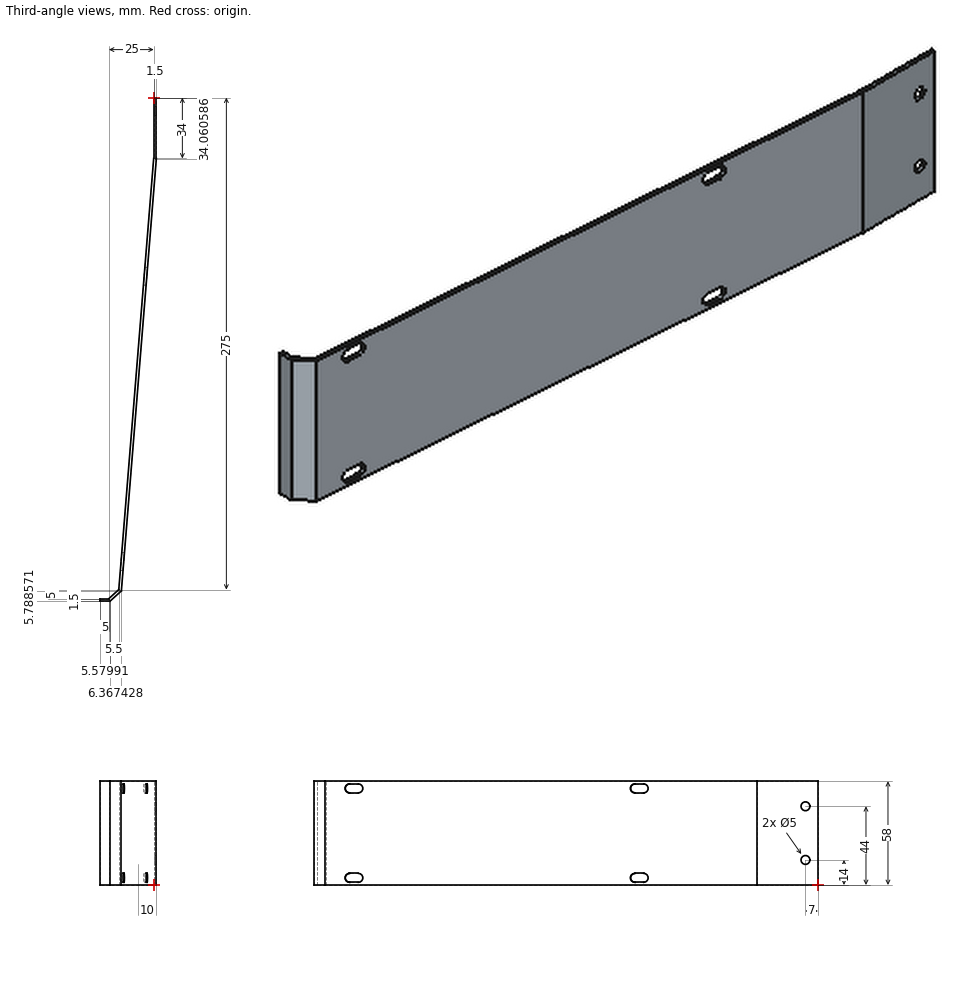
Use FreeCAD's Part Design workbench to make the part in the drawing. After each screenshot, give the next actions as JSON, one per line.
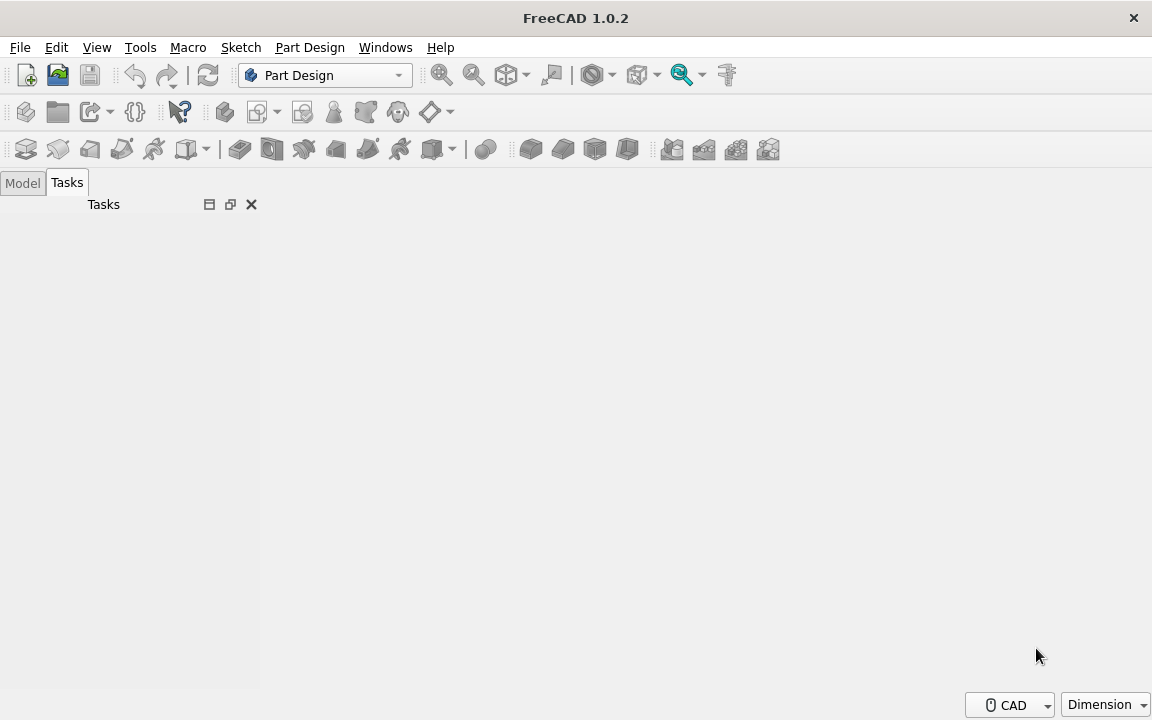
{"action": "left_click", "coordinate": [26, 76]}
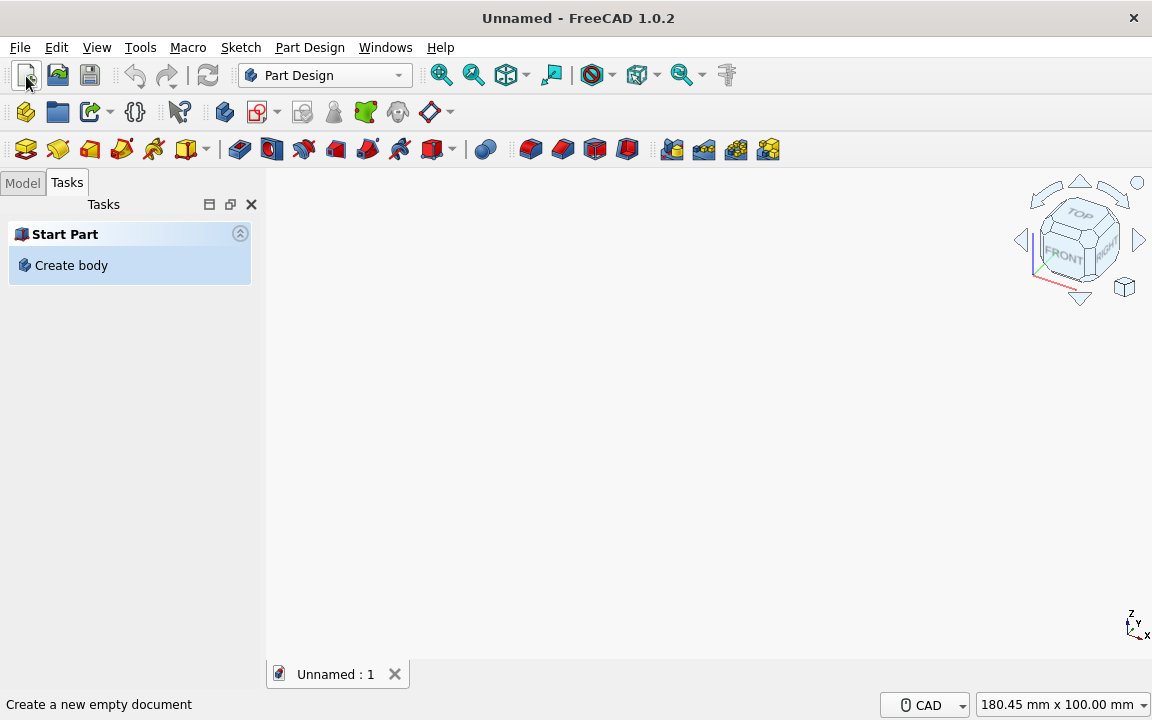
{"action": "left_click", "coordinate": [258, 112]}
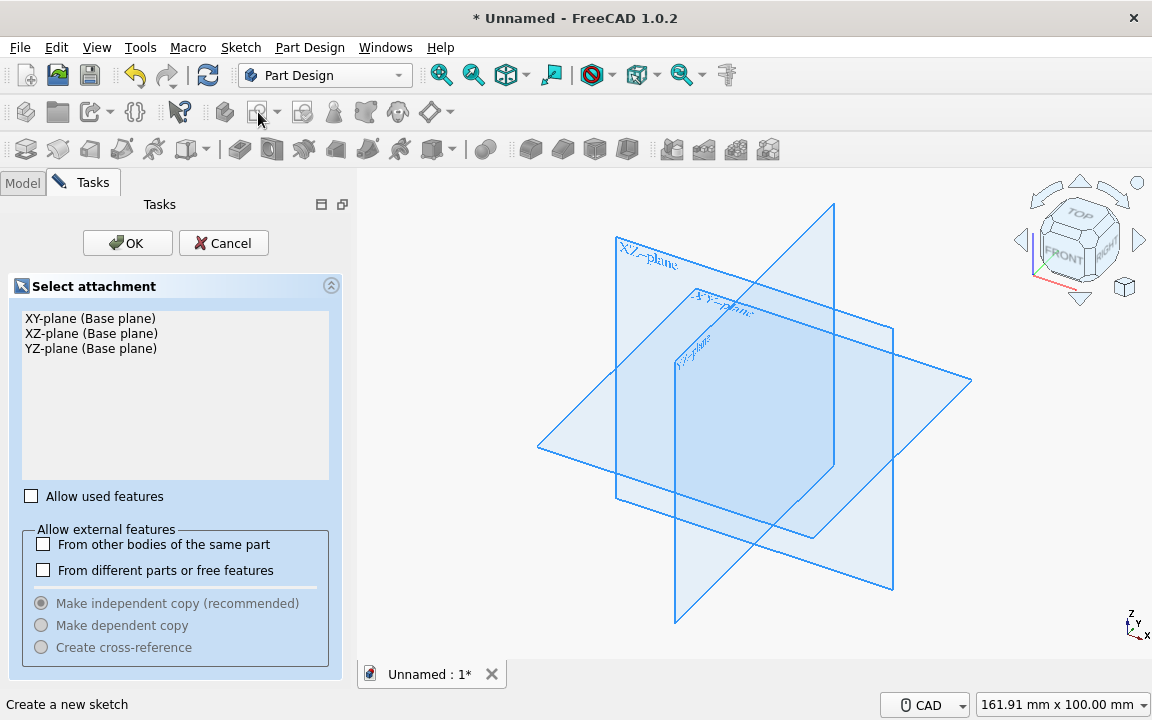
{"action": "left_click", "coordinate": [82, 318]}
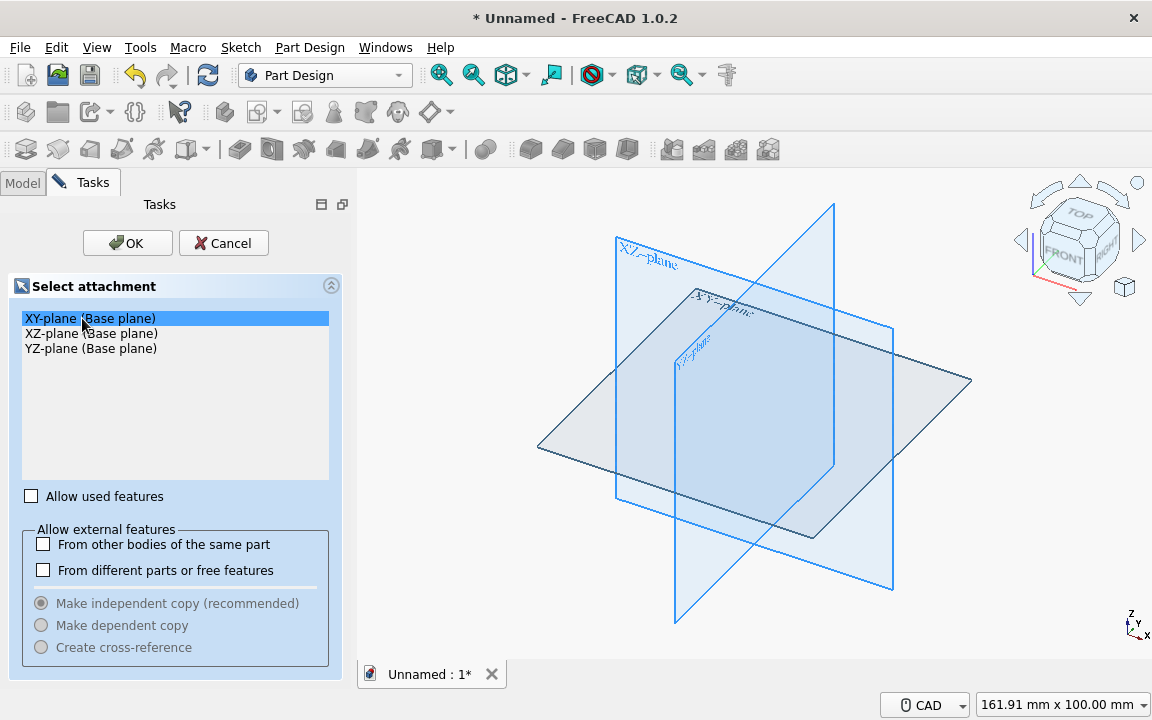
{"action": "left_click", "coordinate": [128, 243]}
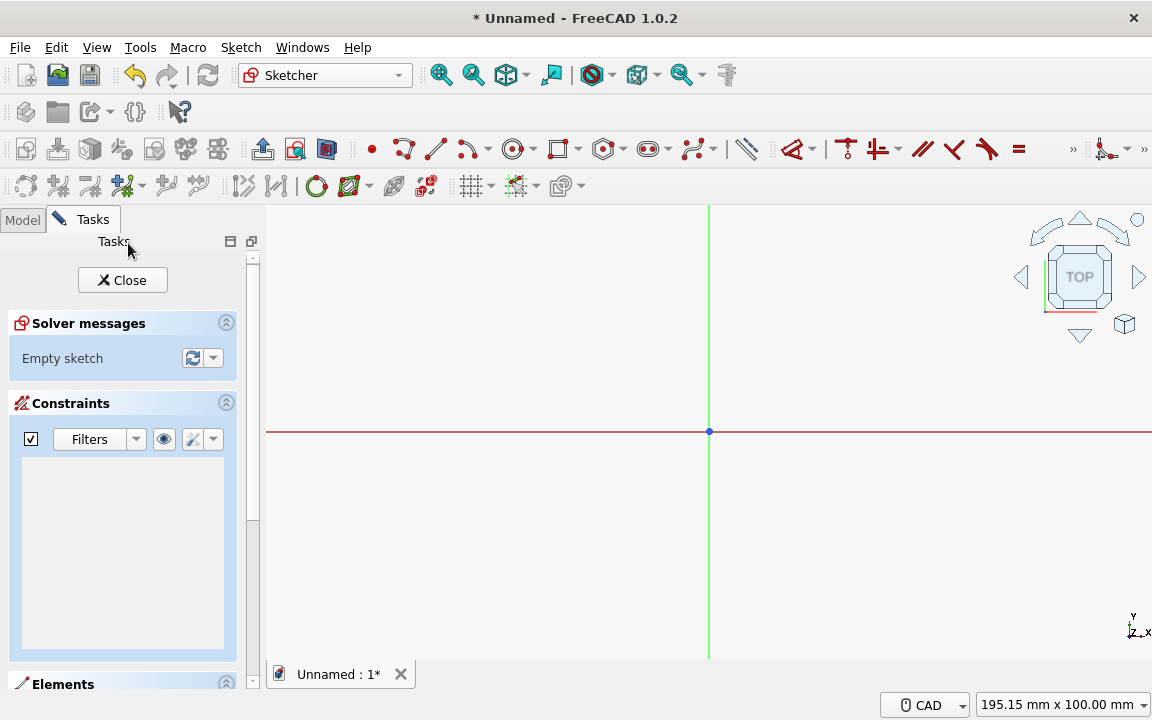
{"action": "scroll", "coordinate": [640, 270], "scroll_direction": "down", "scroll_amount": 8}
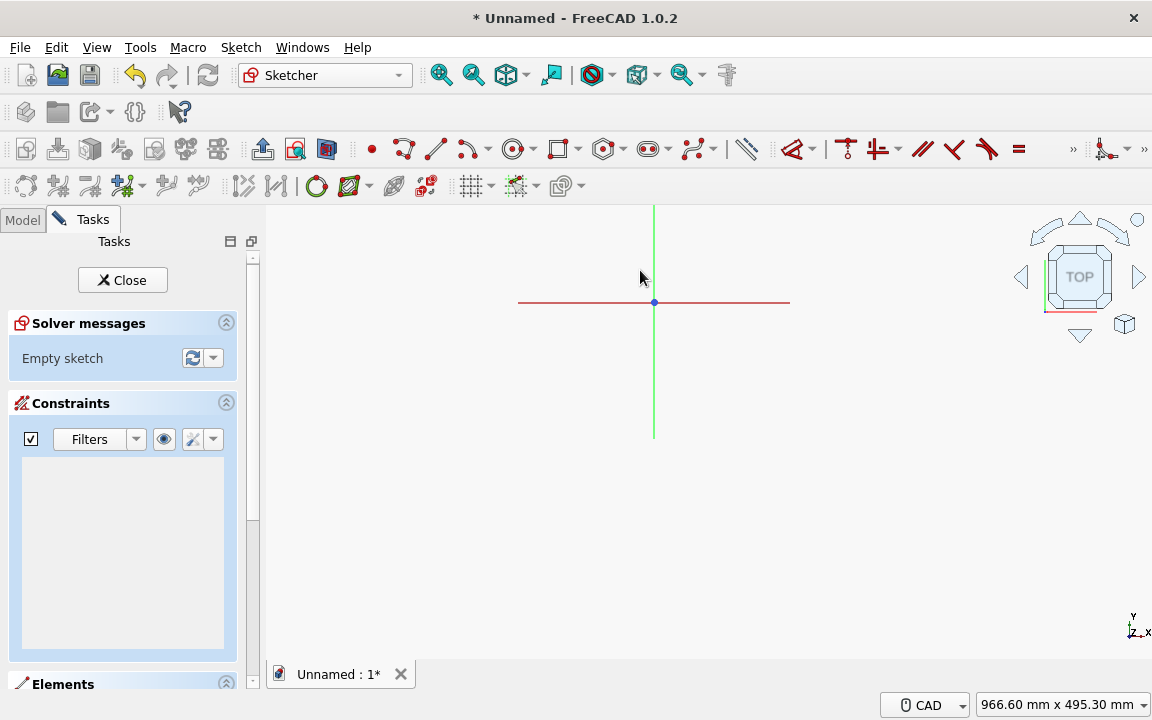
{"action": "left_click", "coordinate": [404, 150]}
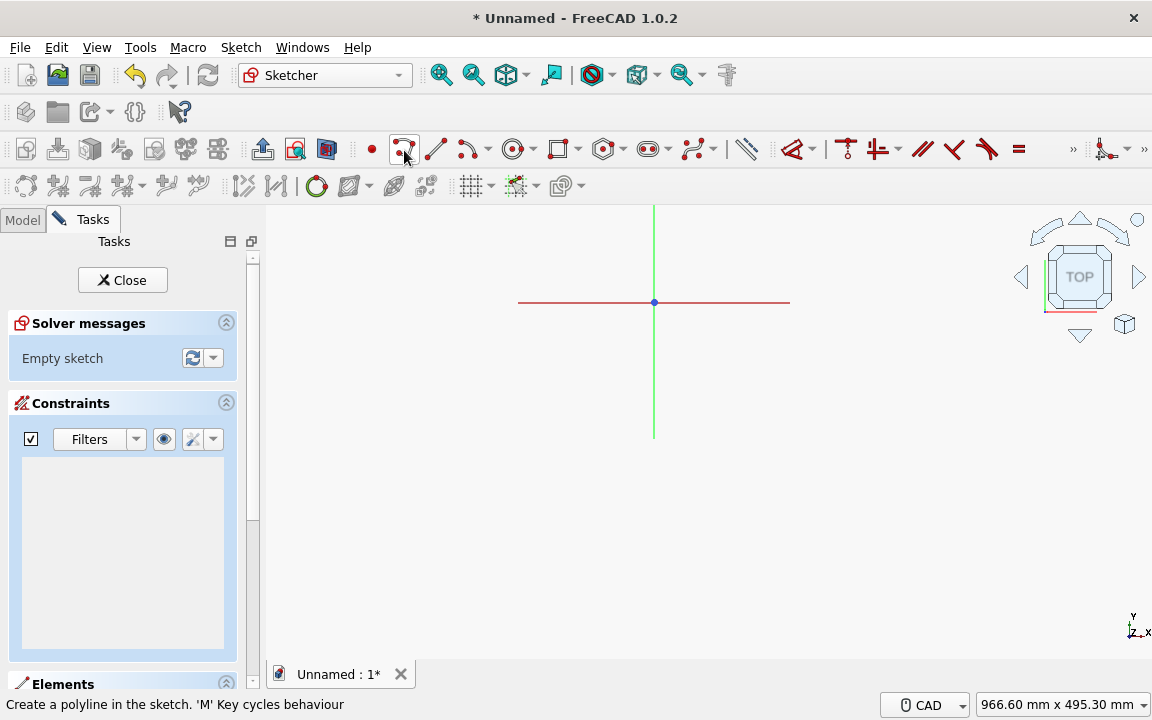
{"action": "left_click", "coordinate": [654, 303]}
{"action": "left_click", "coordinate": [645, 334]}
{"action": "left_click", "coordinate": [636, 555]}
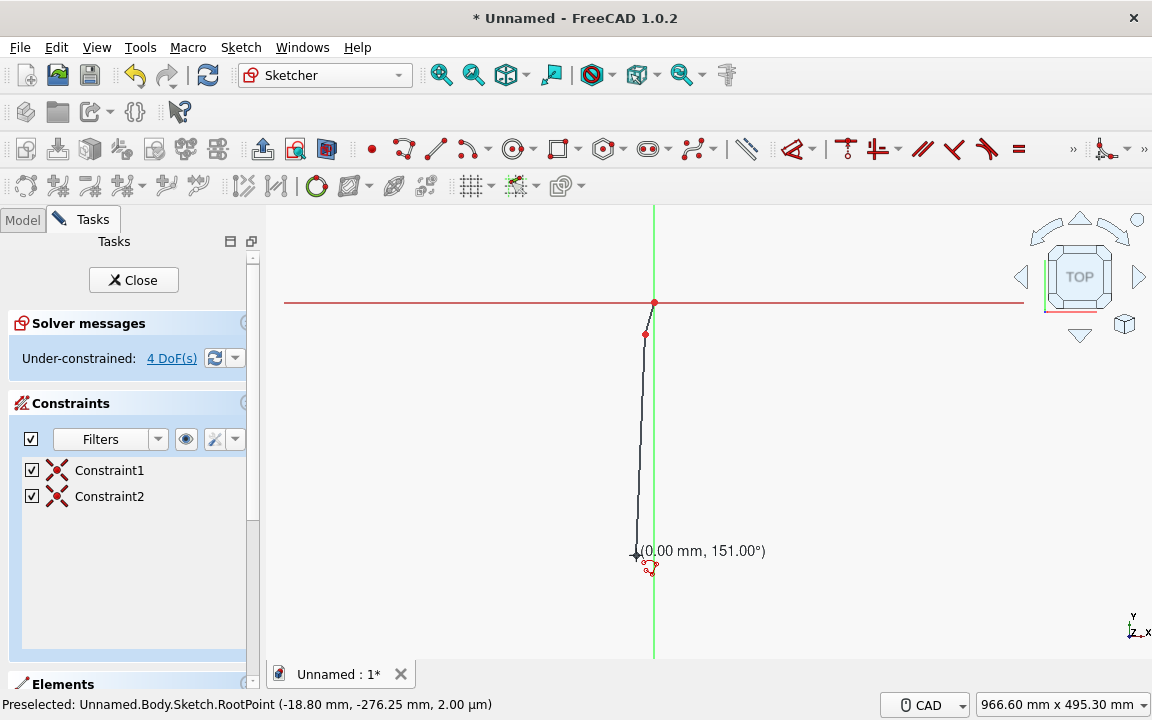
{"action": "scroll", "coordinate": [631, 559], "scroll_direction": "up", "scroll_amount": 5}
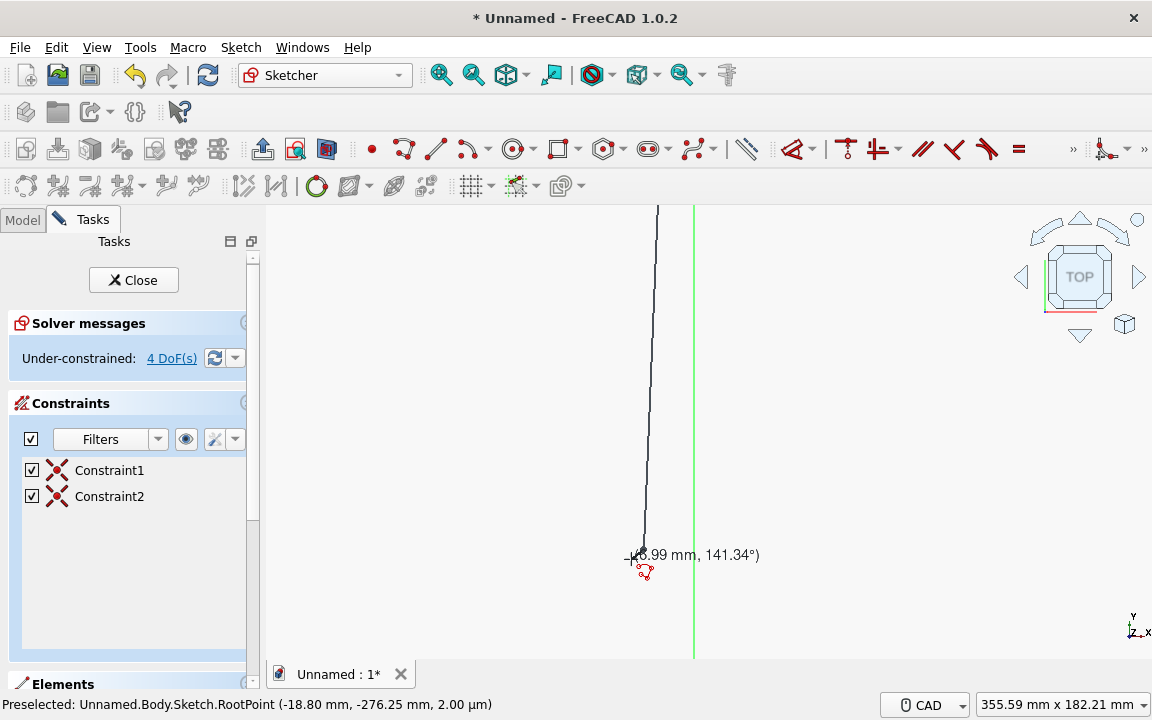
{"action": "left_click", "coordinate": [631, 559]}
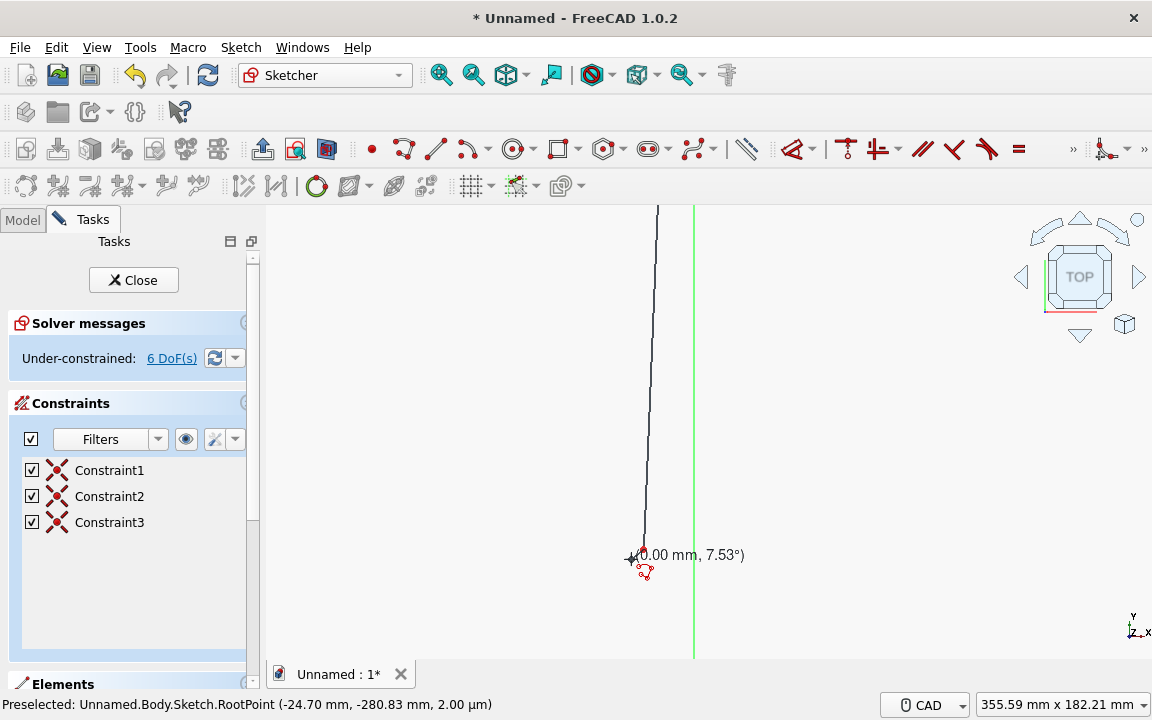
{"action": "scroll", "coordinate": [619, 559], "scroll_direction": "up", "scroll_amount": 2}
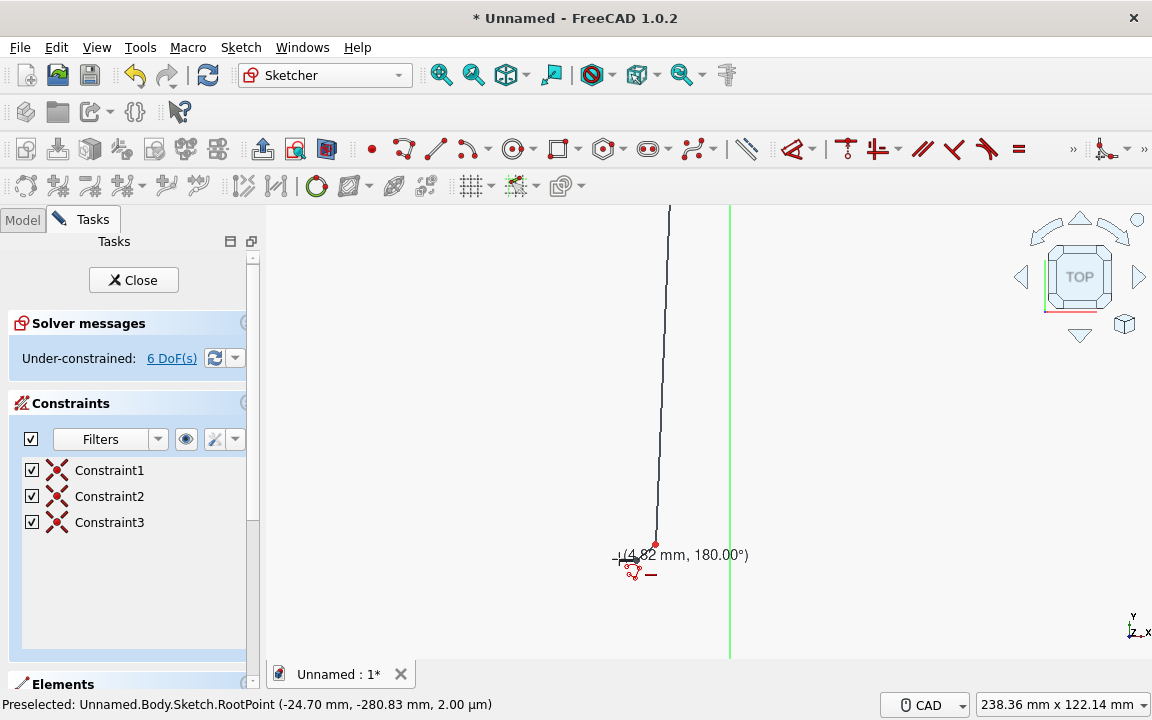
{"action": "left_click", "coordinate": [618, 559]}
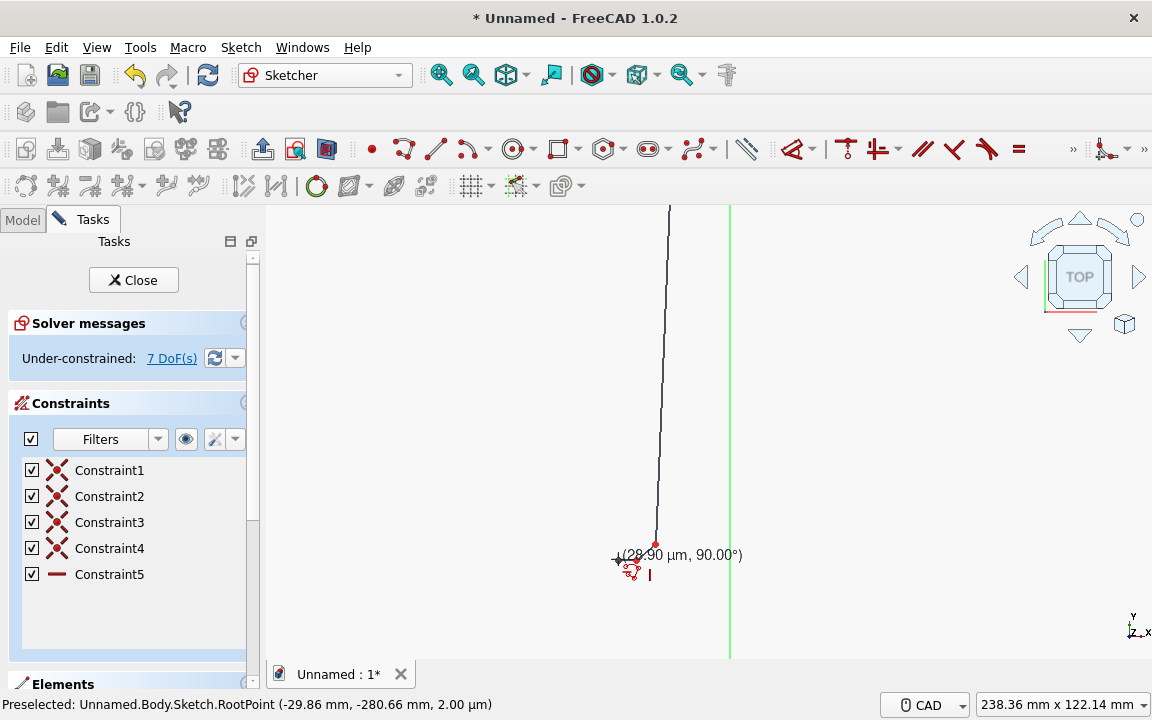
{"action": "scroll", "coordinate": [618, 564], "scroll_direction": "up", "scroll_amount": 6}